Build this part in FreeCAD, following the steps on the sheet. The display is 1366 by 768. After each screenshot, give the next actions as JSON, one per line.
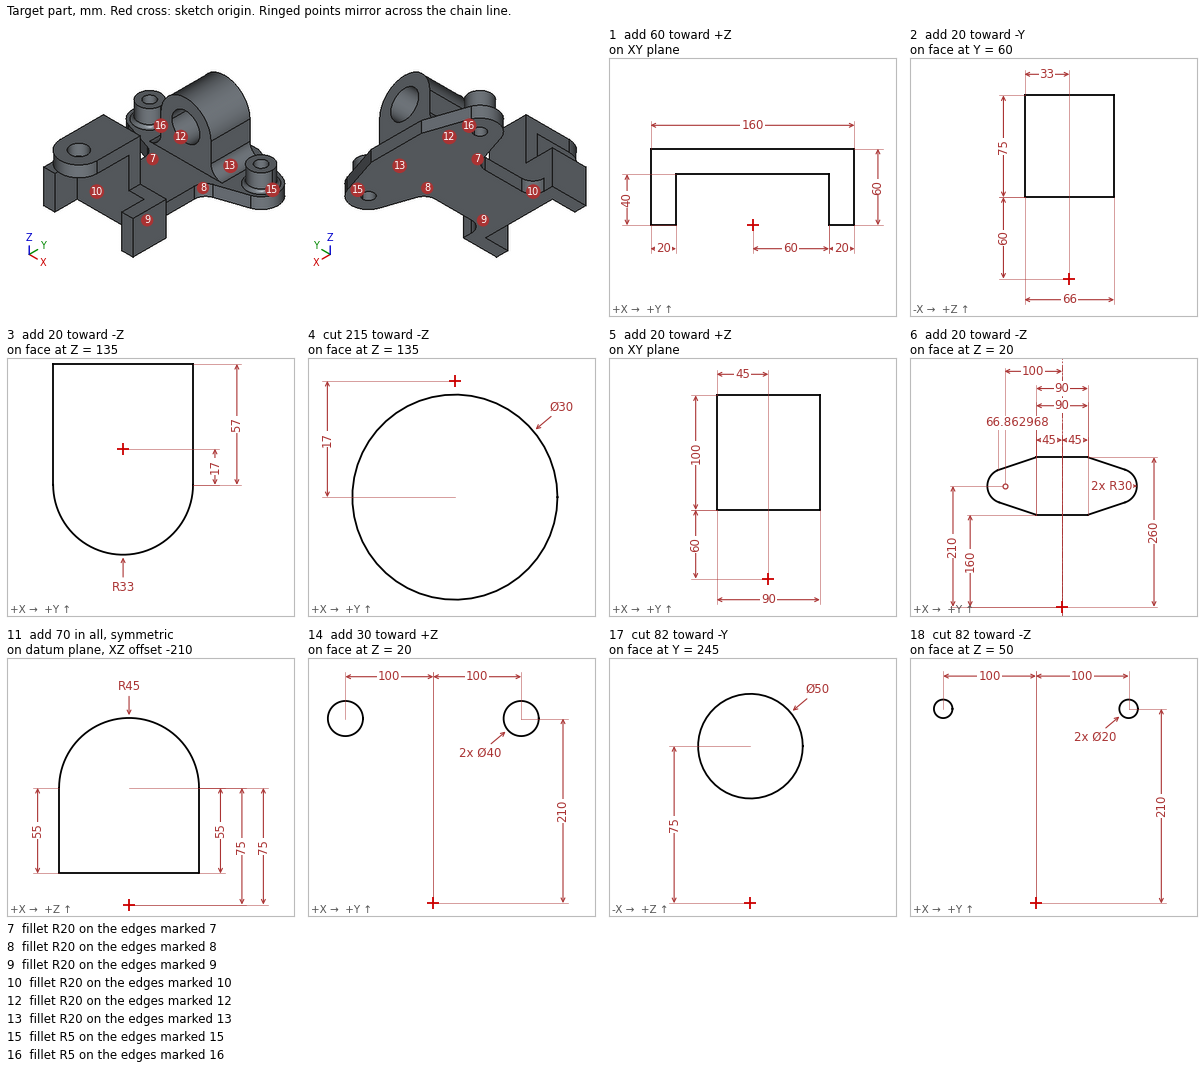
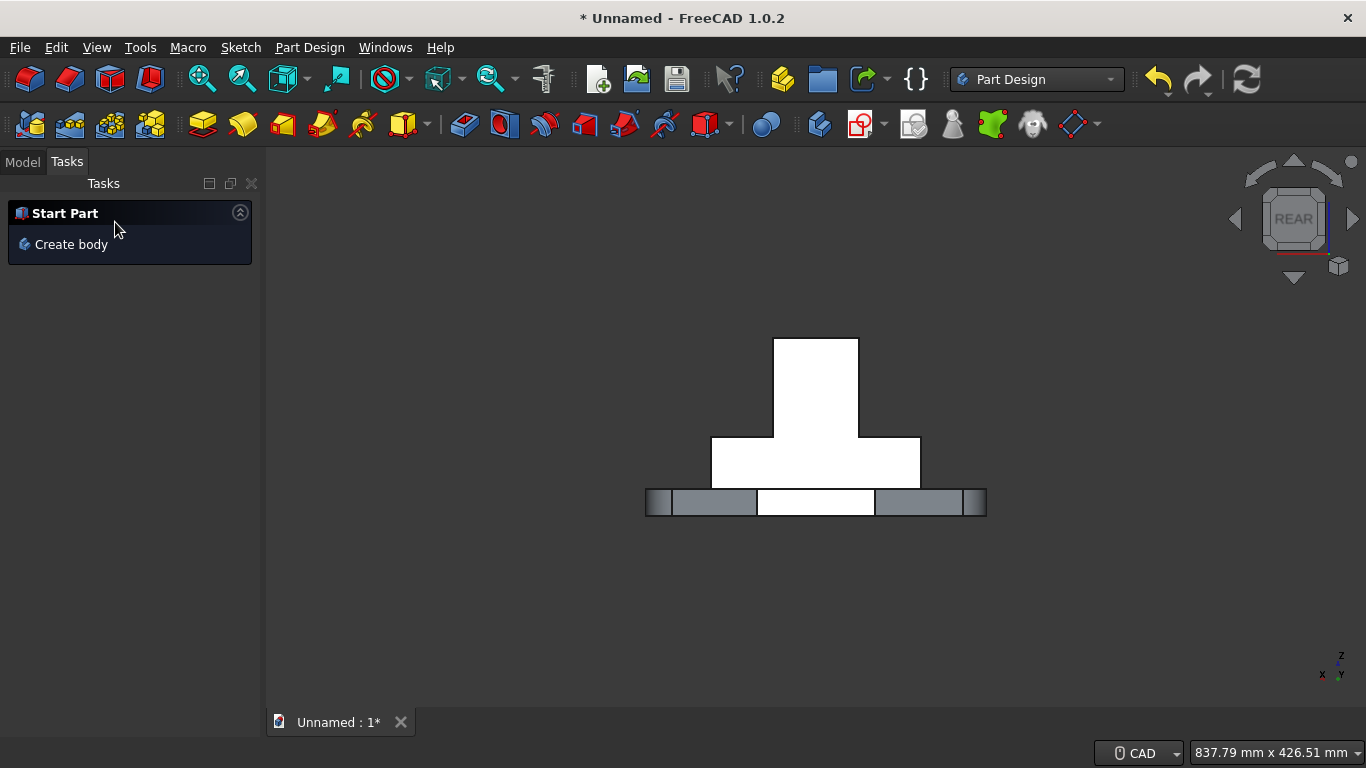
{"action": "key", "text": "6"}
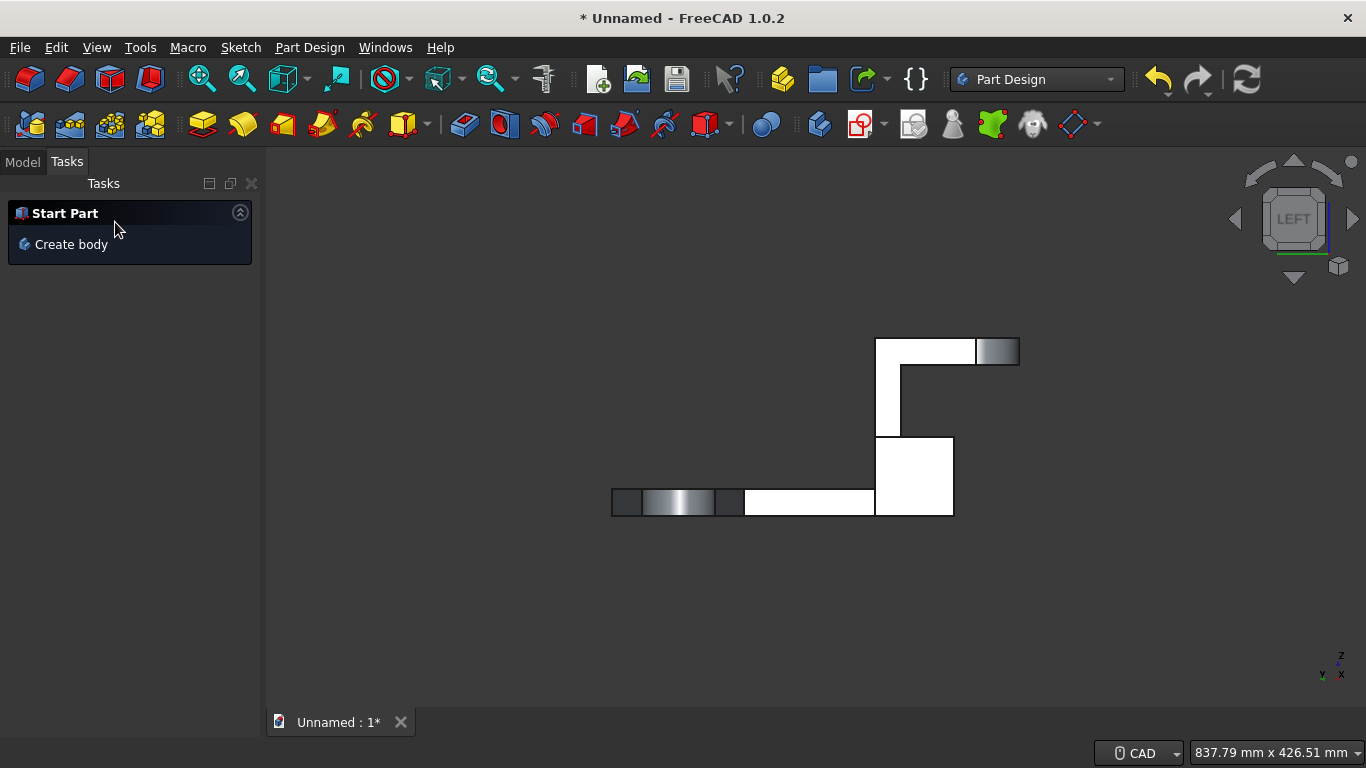
{"action": "key", "text": "v f"}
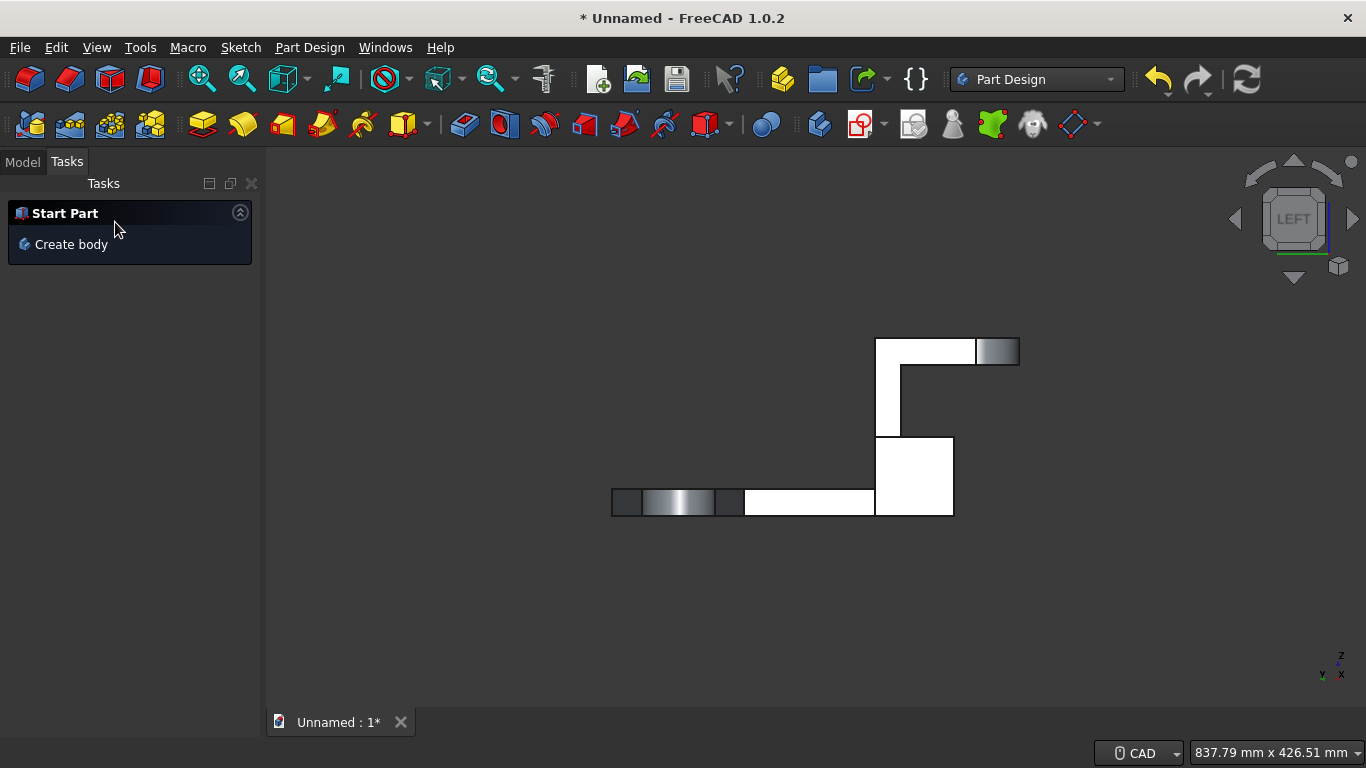
{"action": "key", "text": "v 3"}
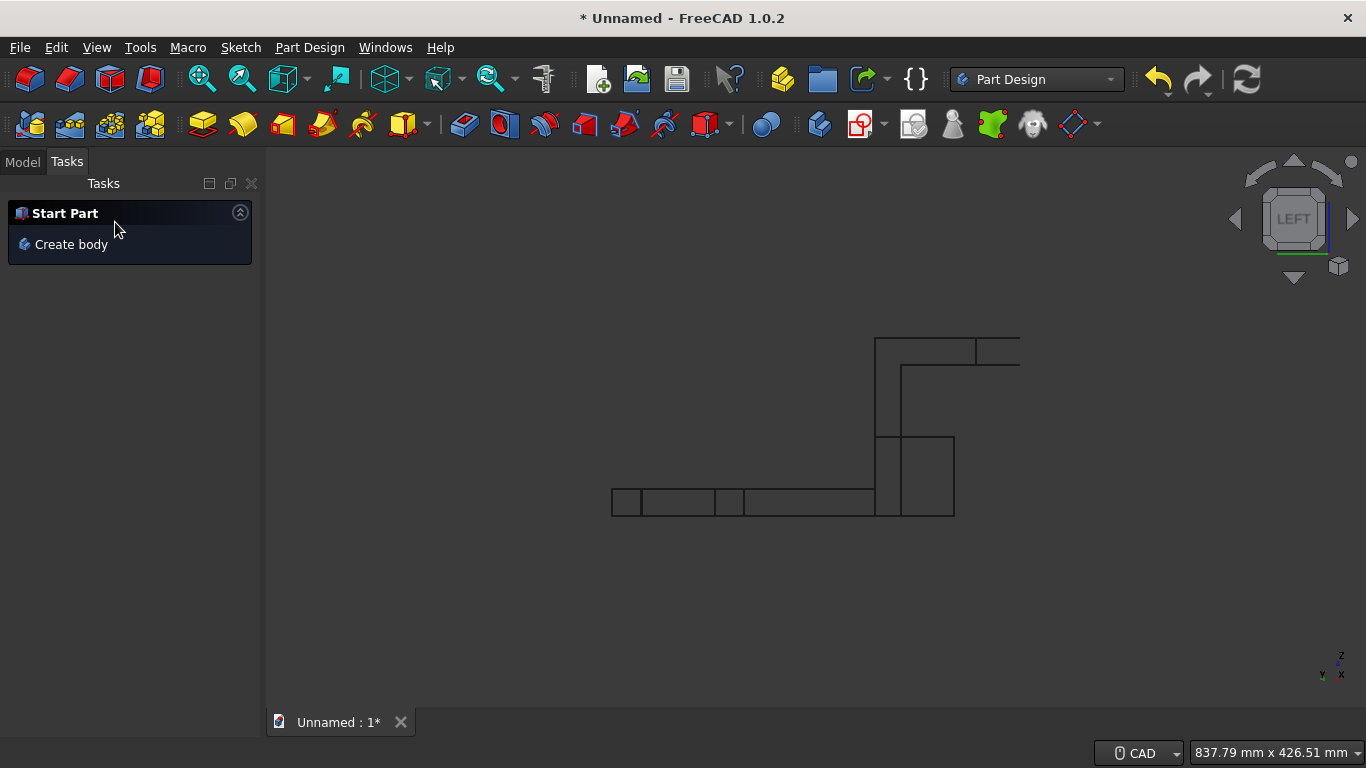
{"action": "key", "text": "0"}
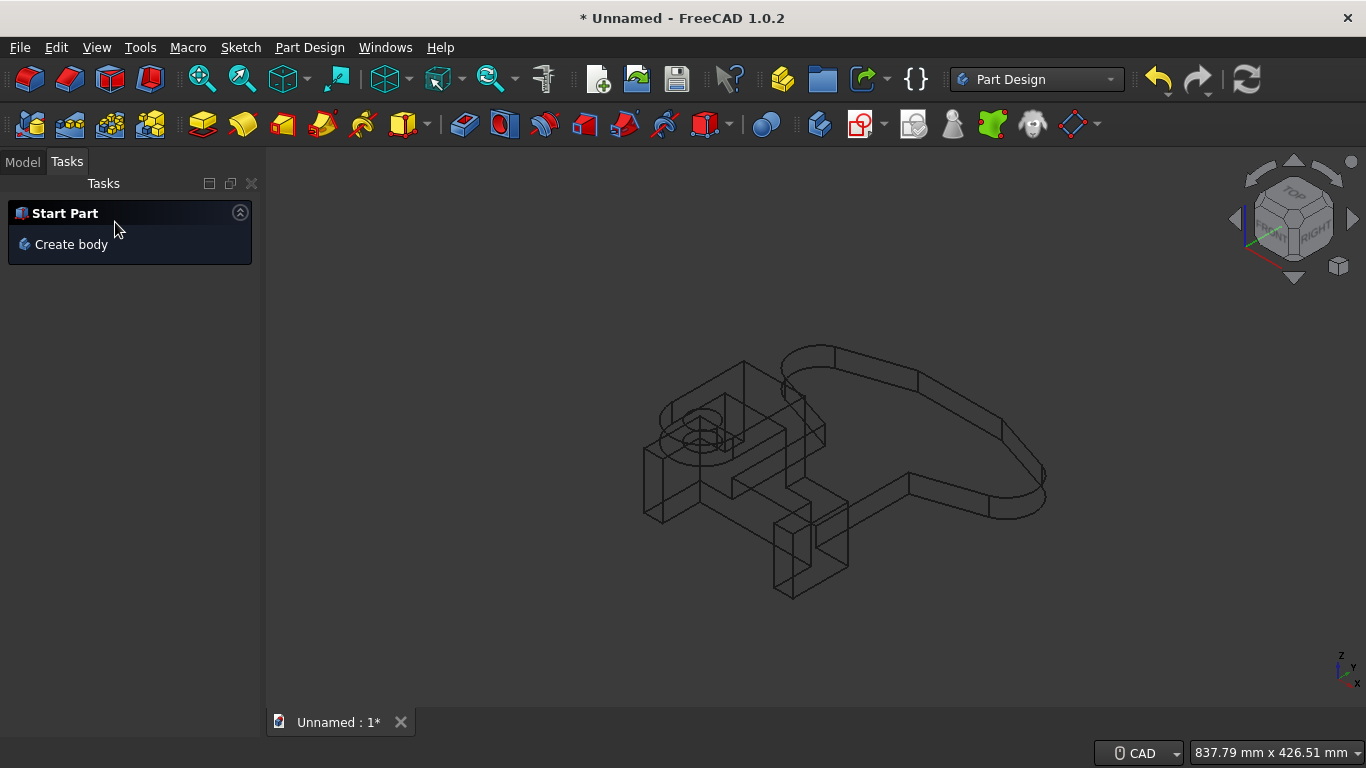
{"action": "left_click", "coordinate": [825, 434]}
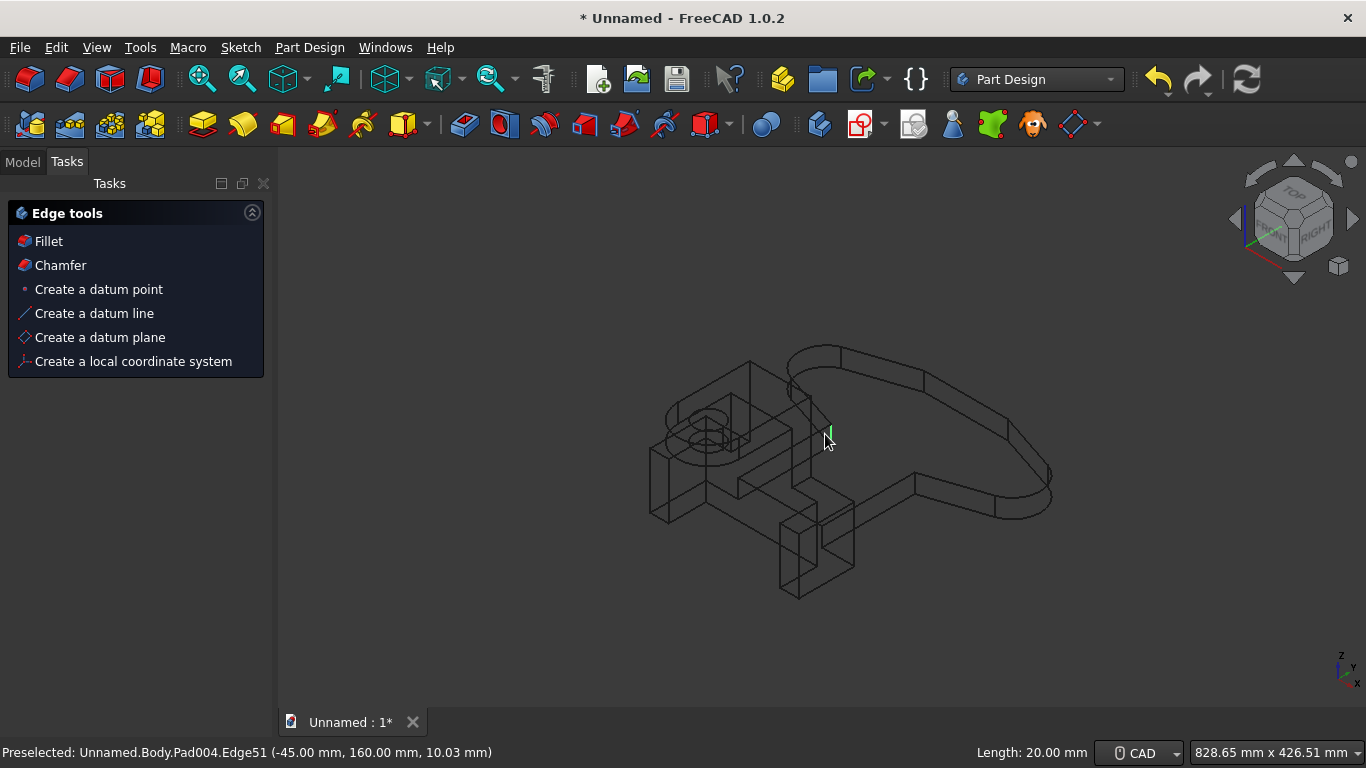
{"action": "key", "text": "v 1"}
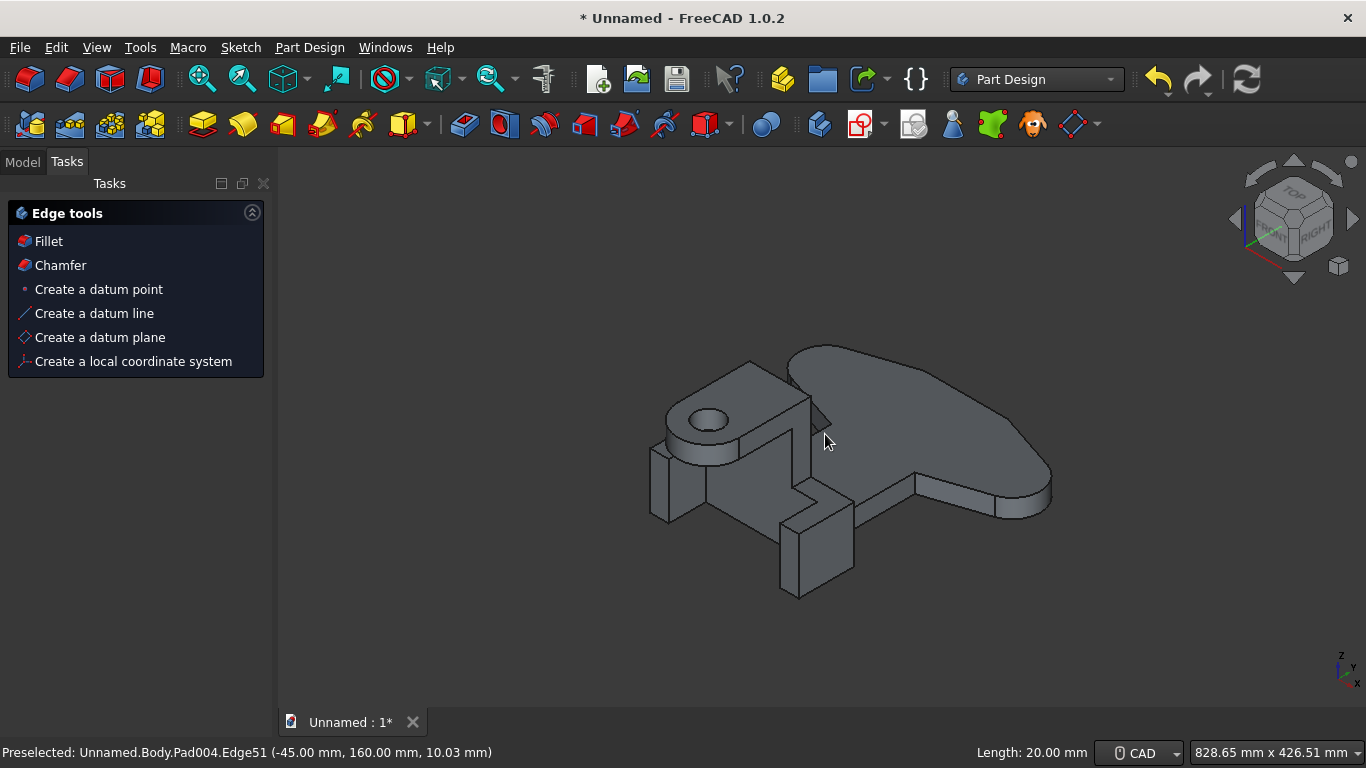
{"action": "left_click", "coordinate": [30, 80]}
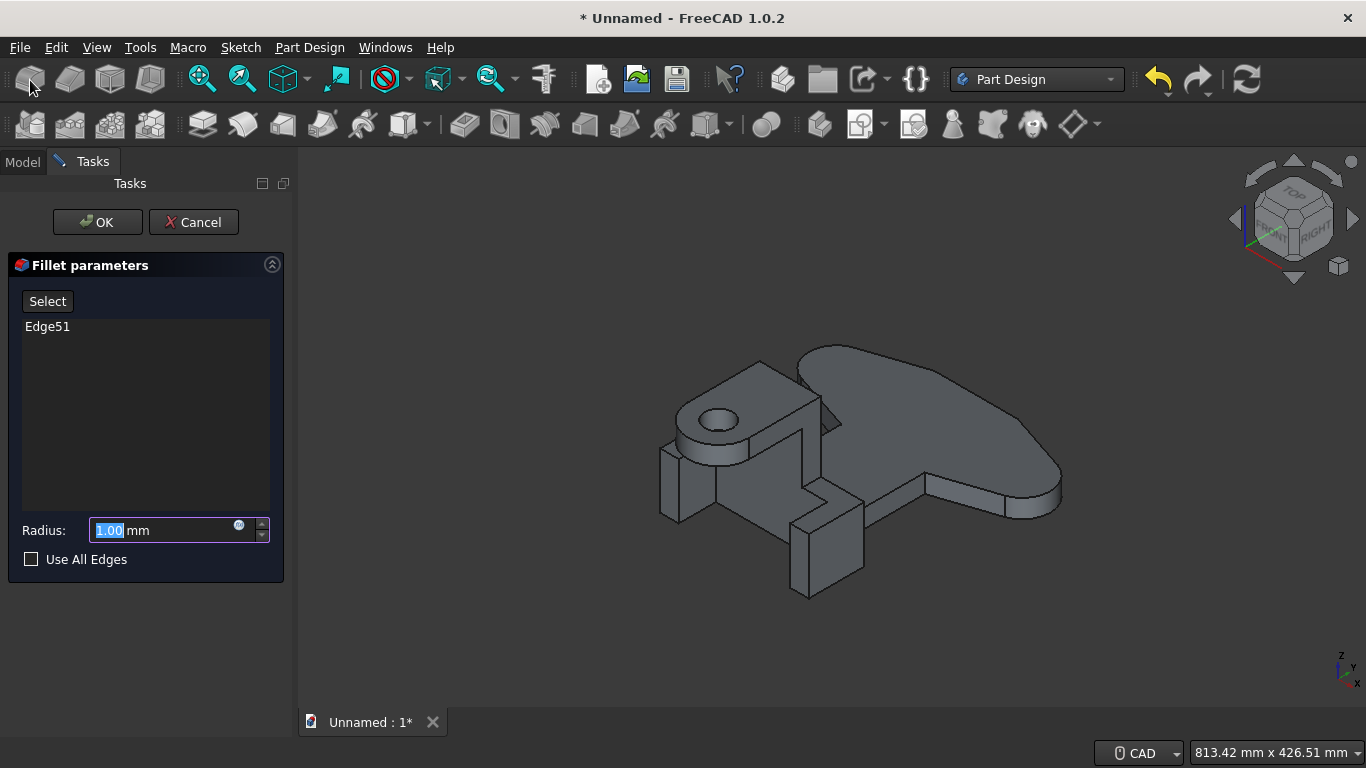
{"action": "type", "text": "20"}
{"action": "key", "text": "Tab"}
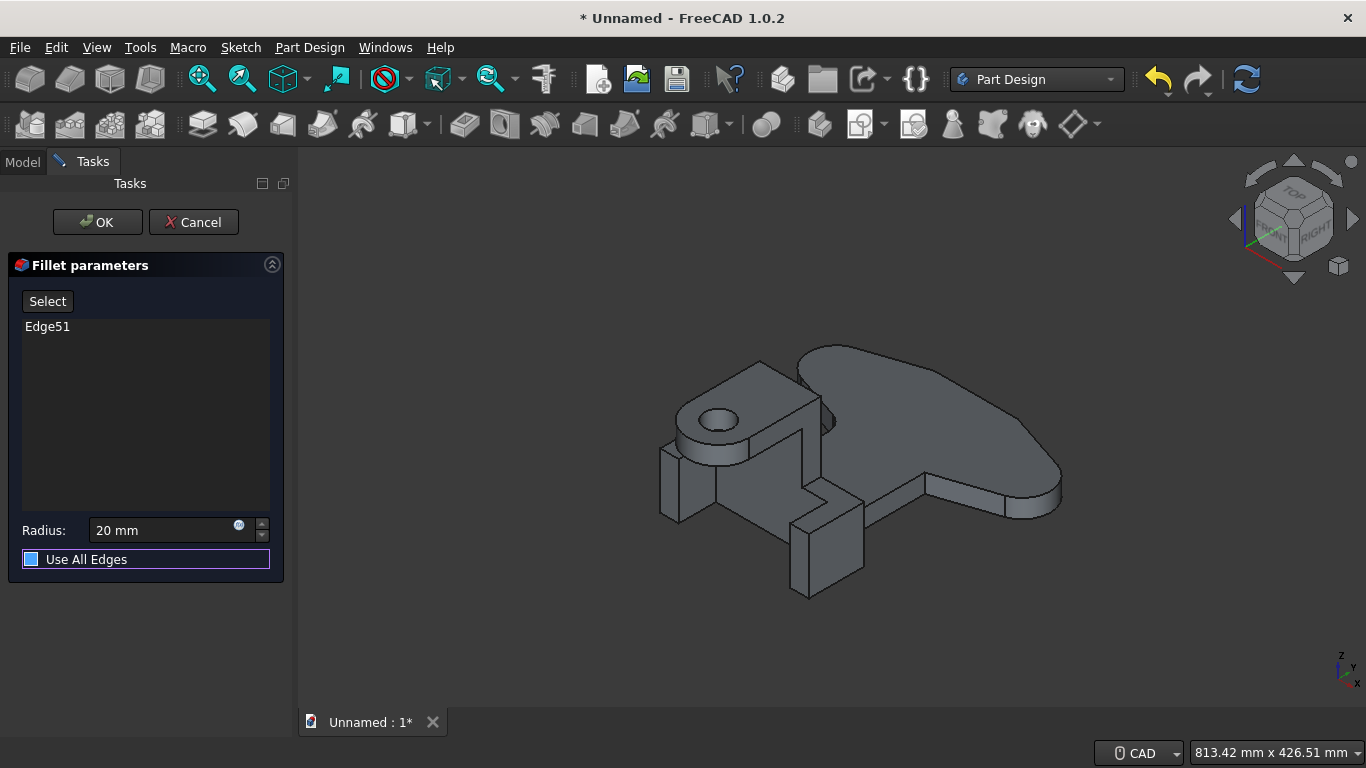
{"action": "left_click", "coordinate": [98, 222]}